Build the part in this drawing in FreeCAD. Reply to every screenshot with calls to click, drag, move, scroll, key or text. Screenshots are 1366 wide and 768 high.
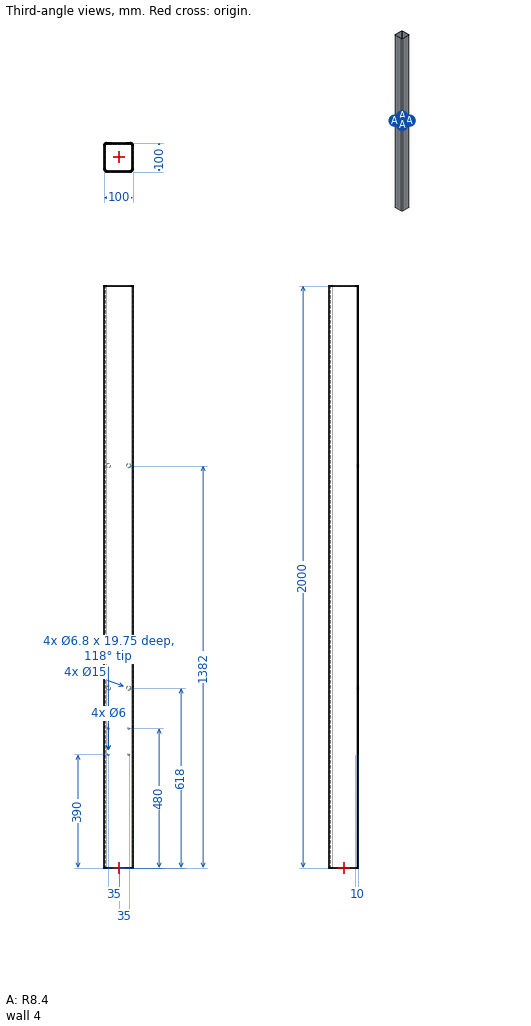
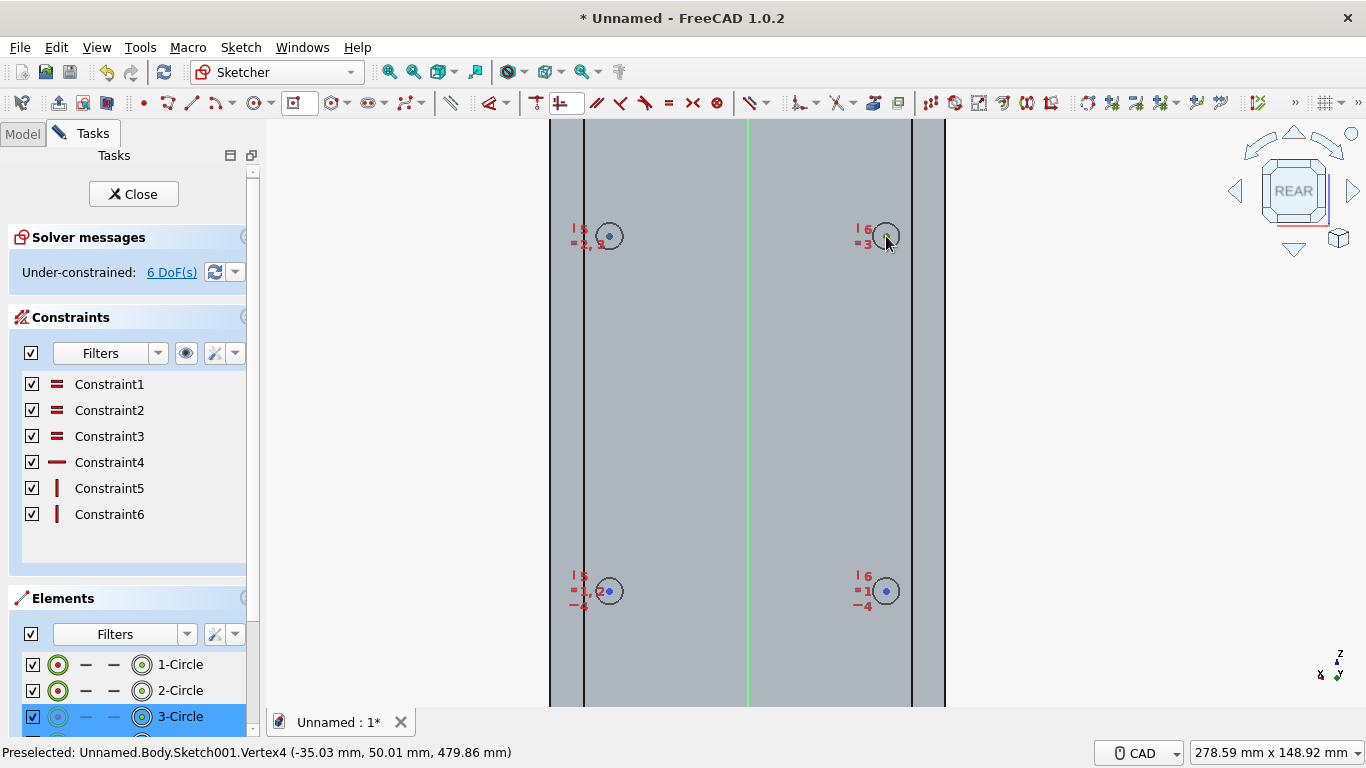
click(578, 104)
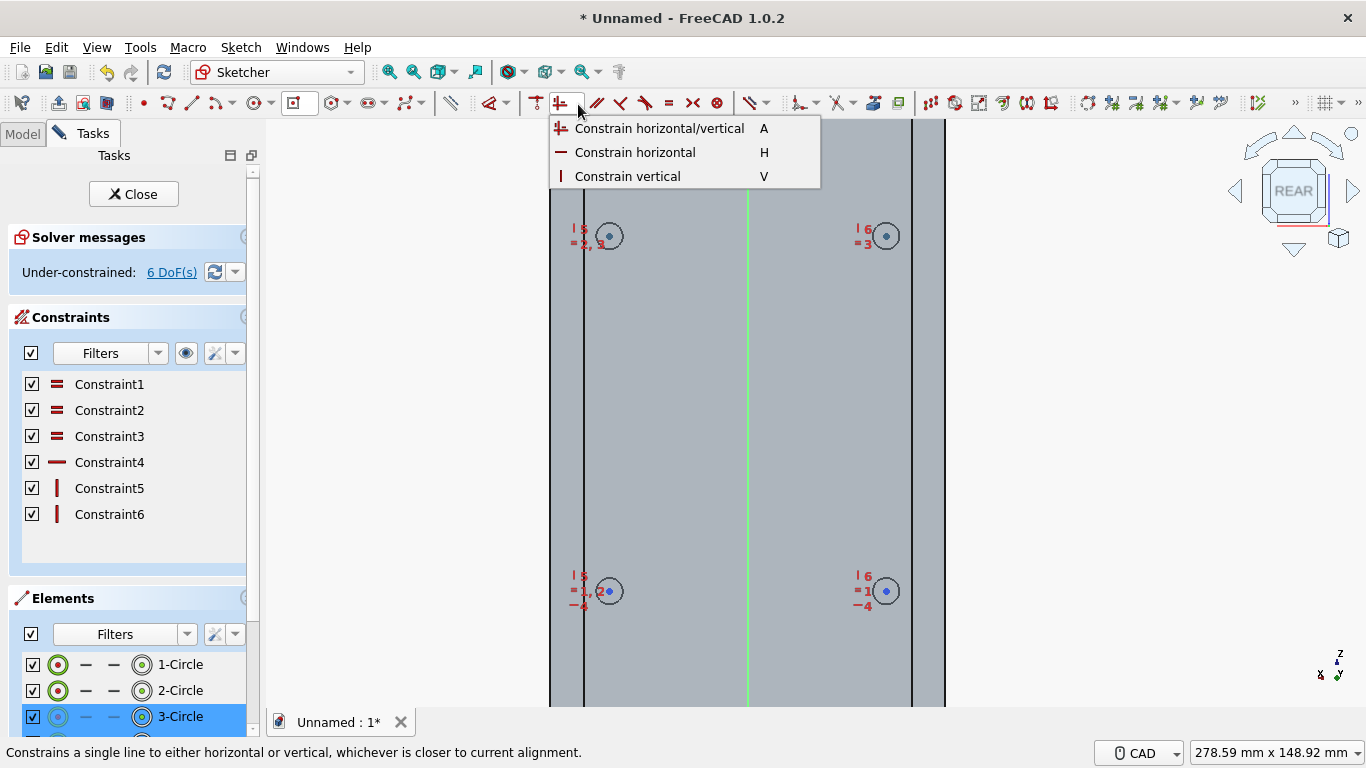
click(685, 152)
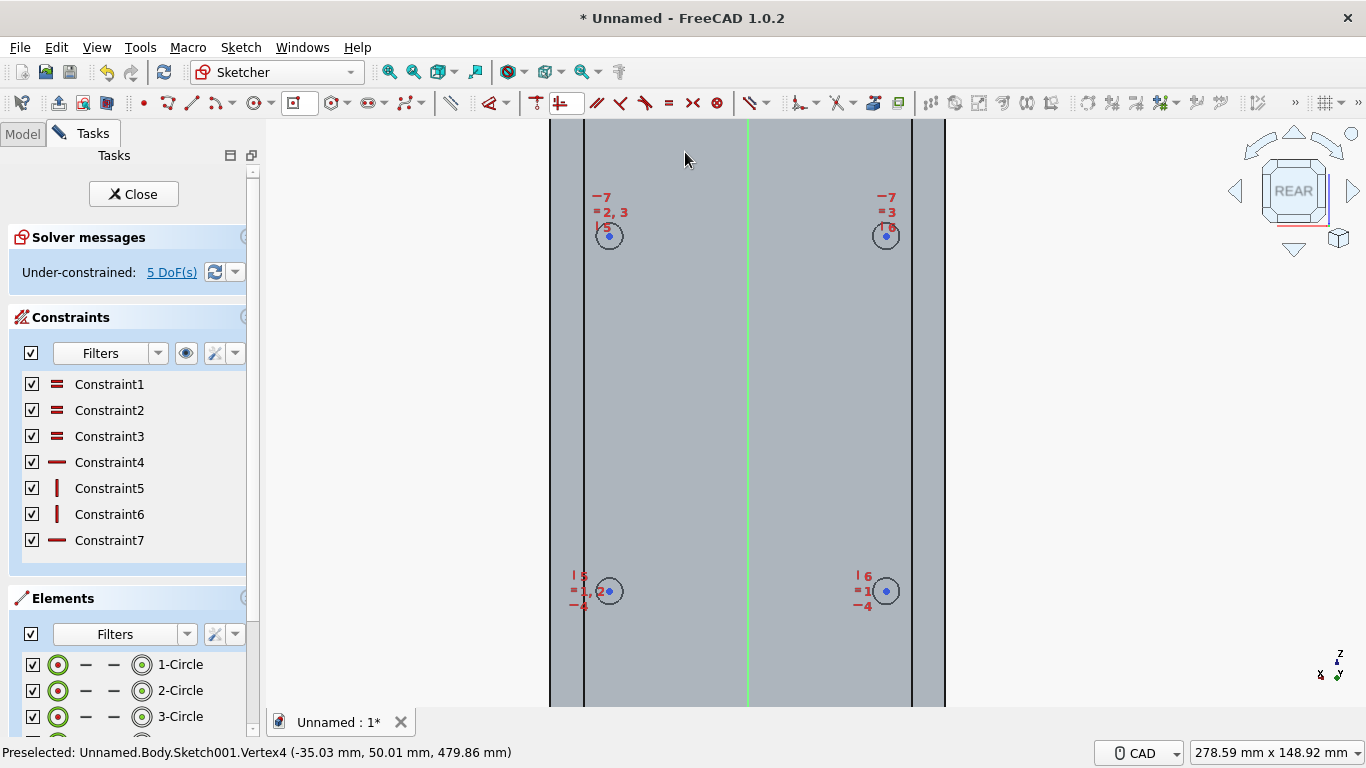
click(490, 104)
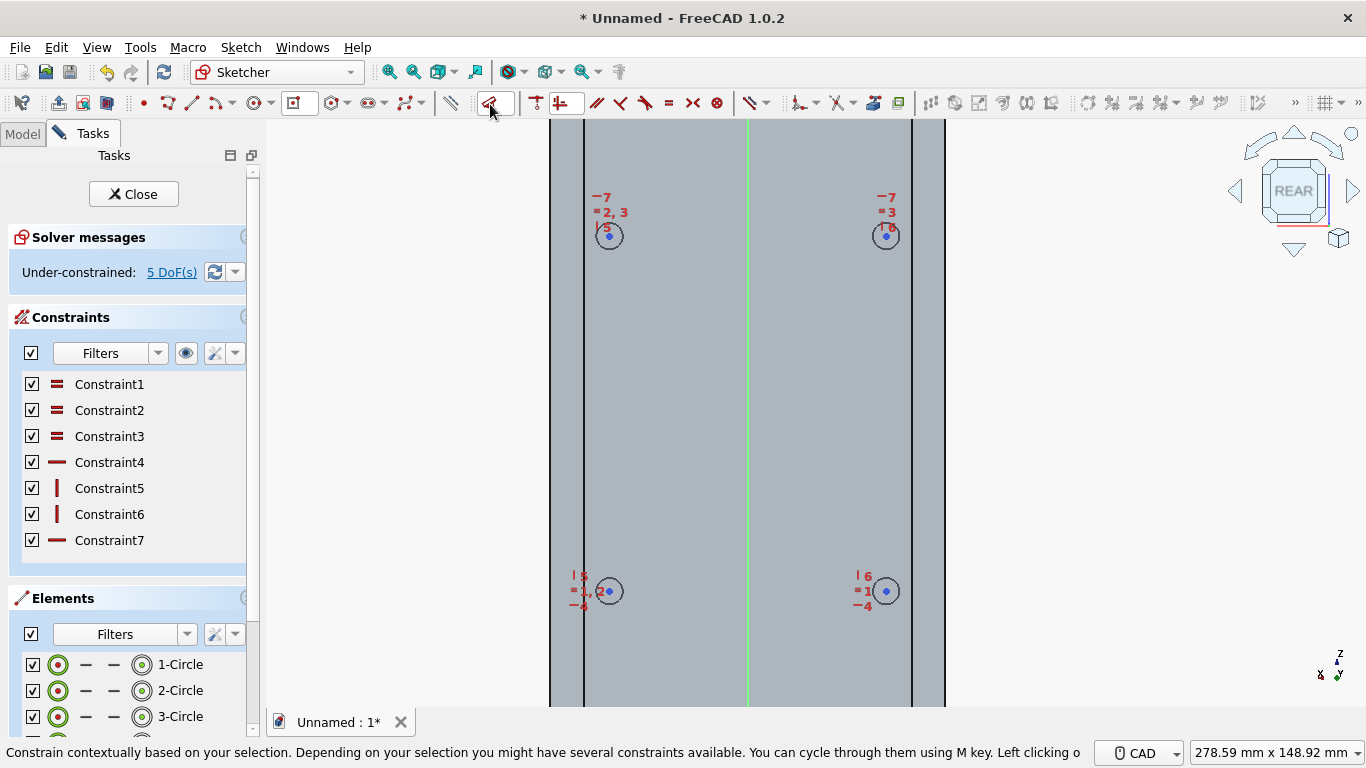
scroll(895, 582, up, 2)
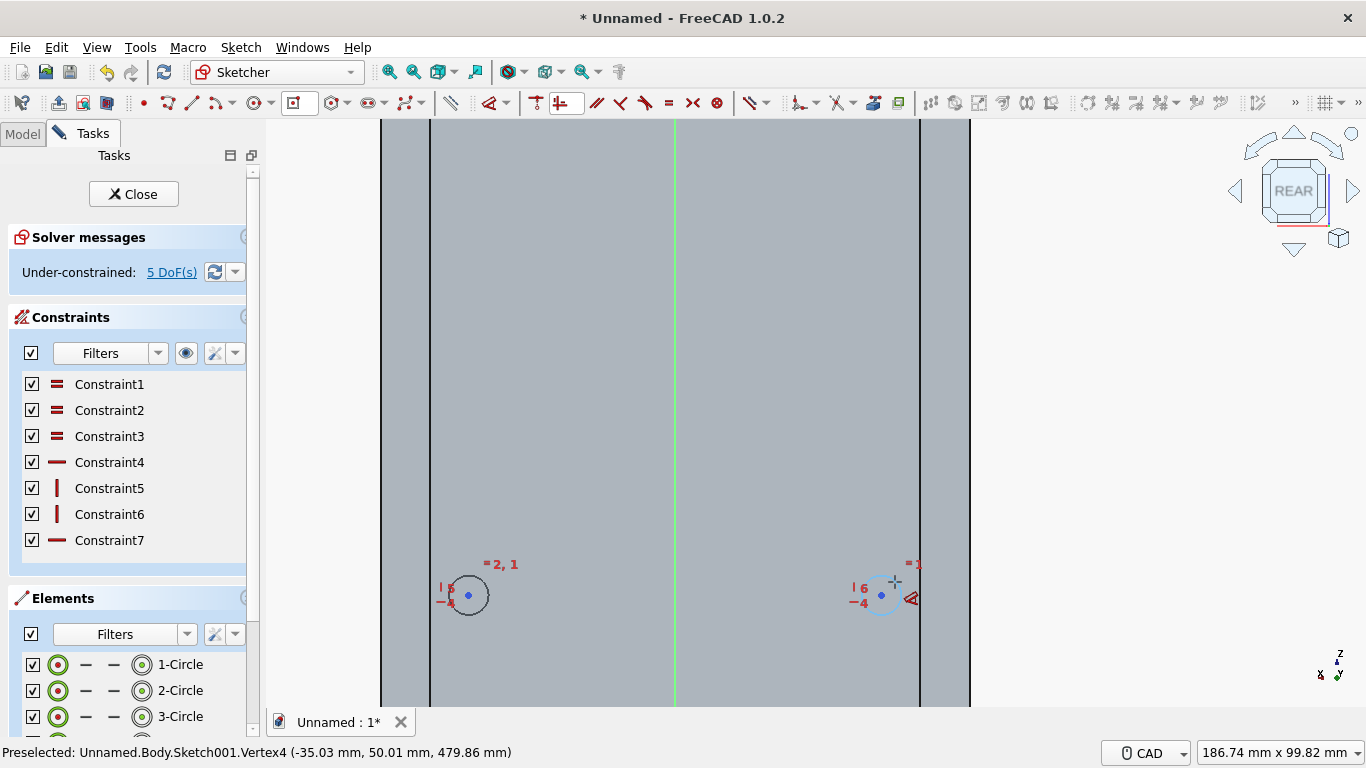
click(895, 581)
click(917, 558)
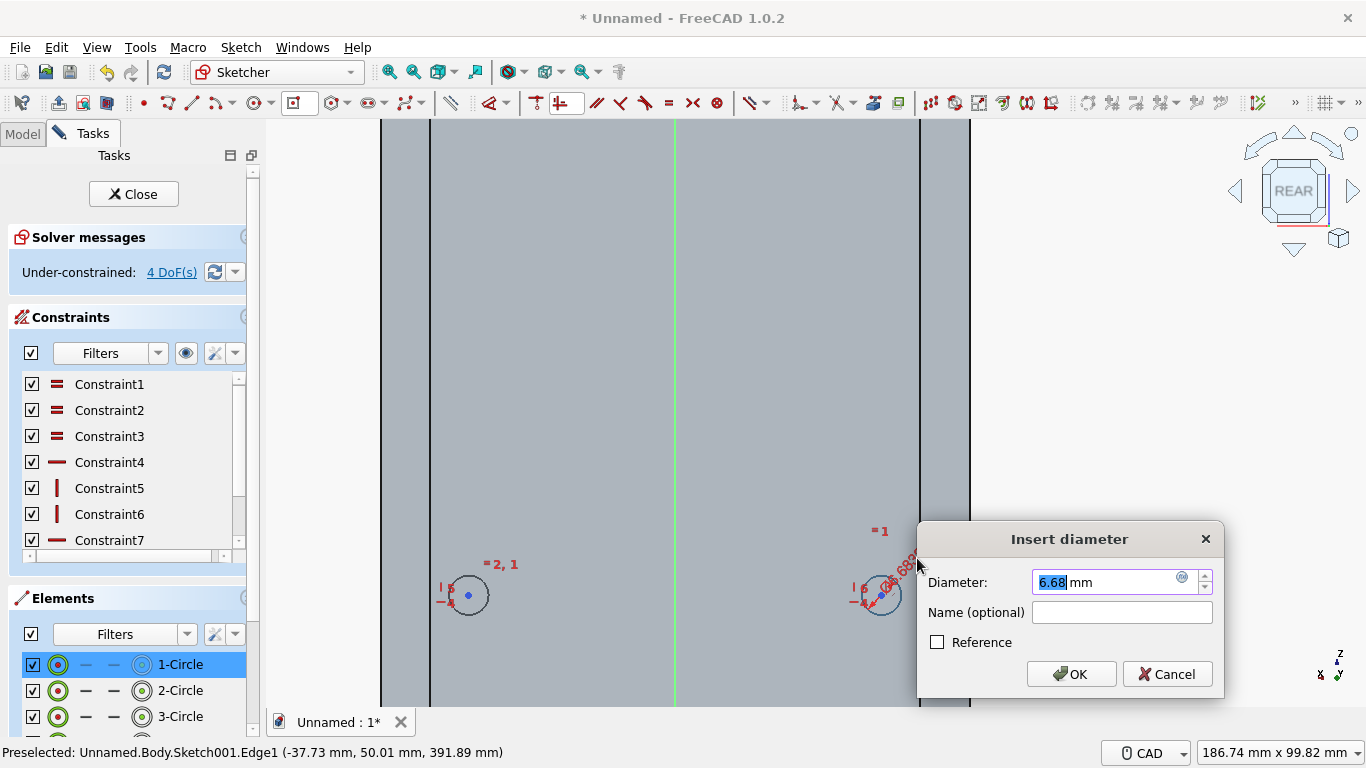
text(6.8)
key(Return)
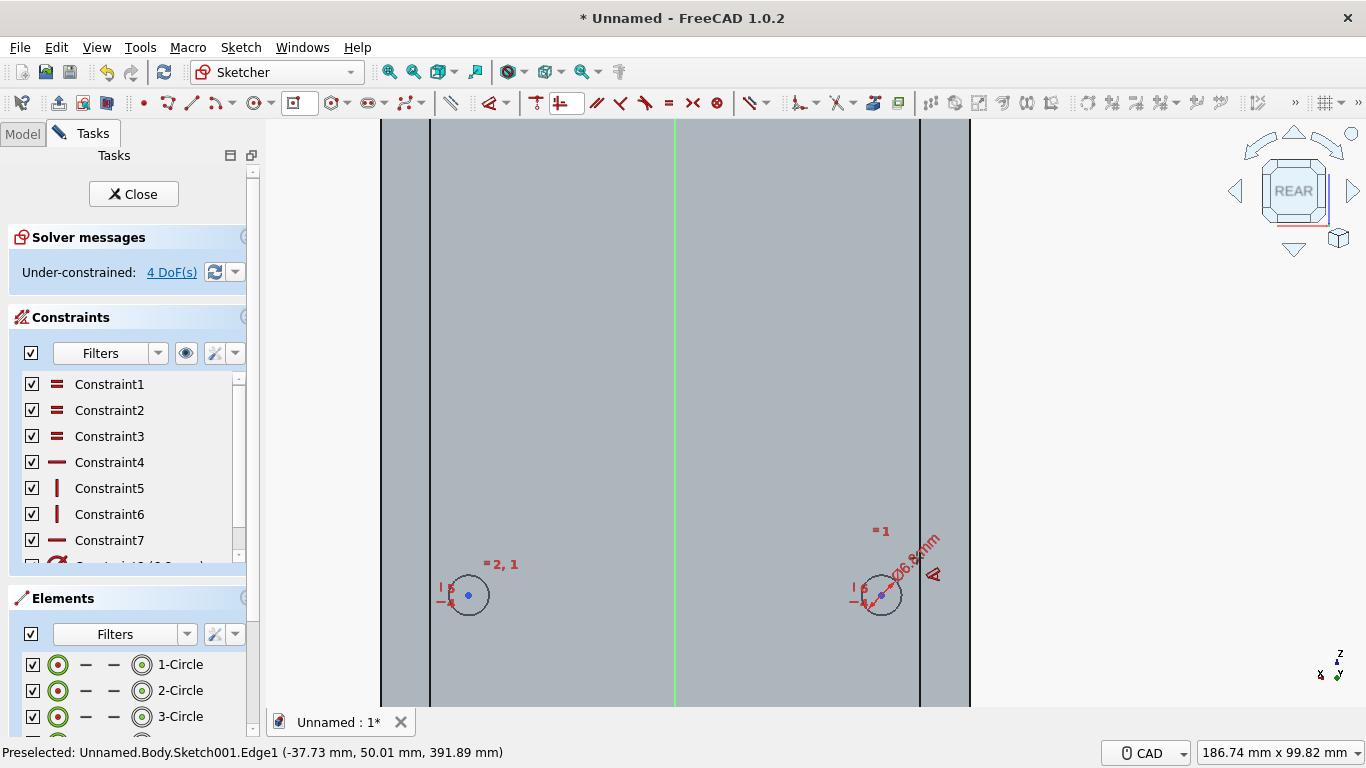
click(882, 595)
click(778, 561)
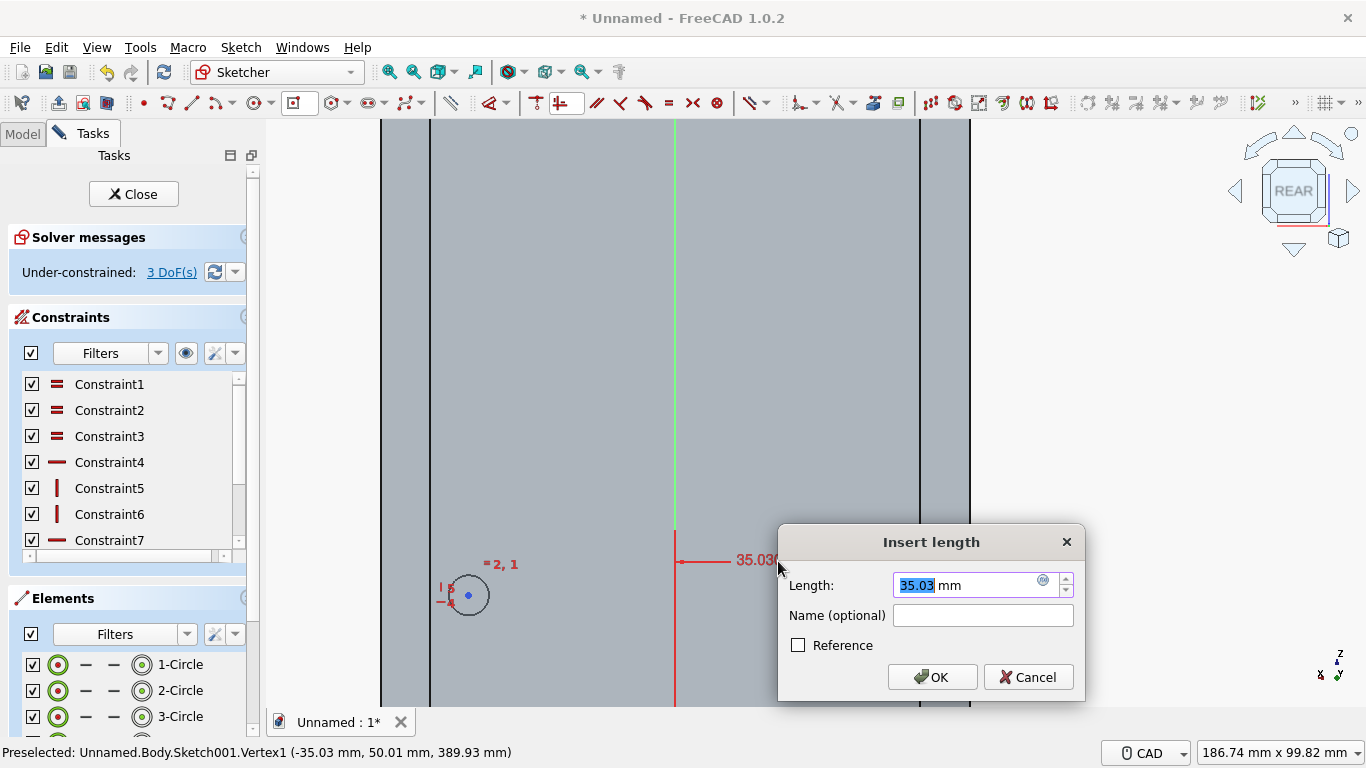
text(35)
key(Return)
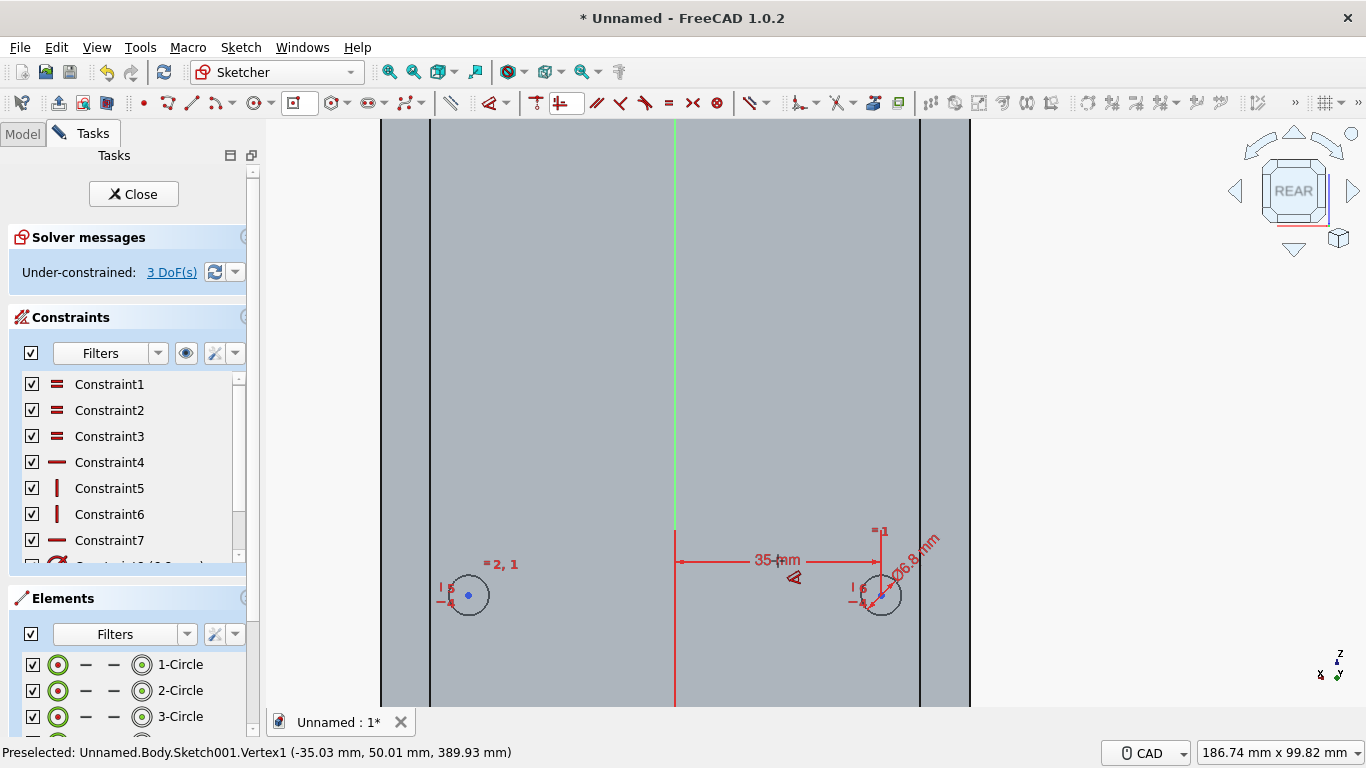
click(469, 595)
click(572, 561)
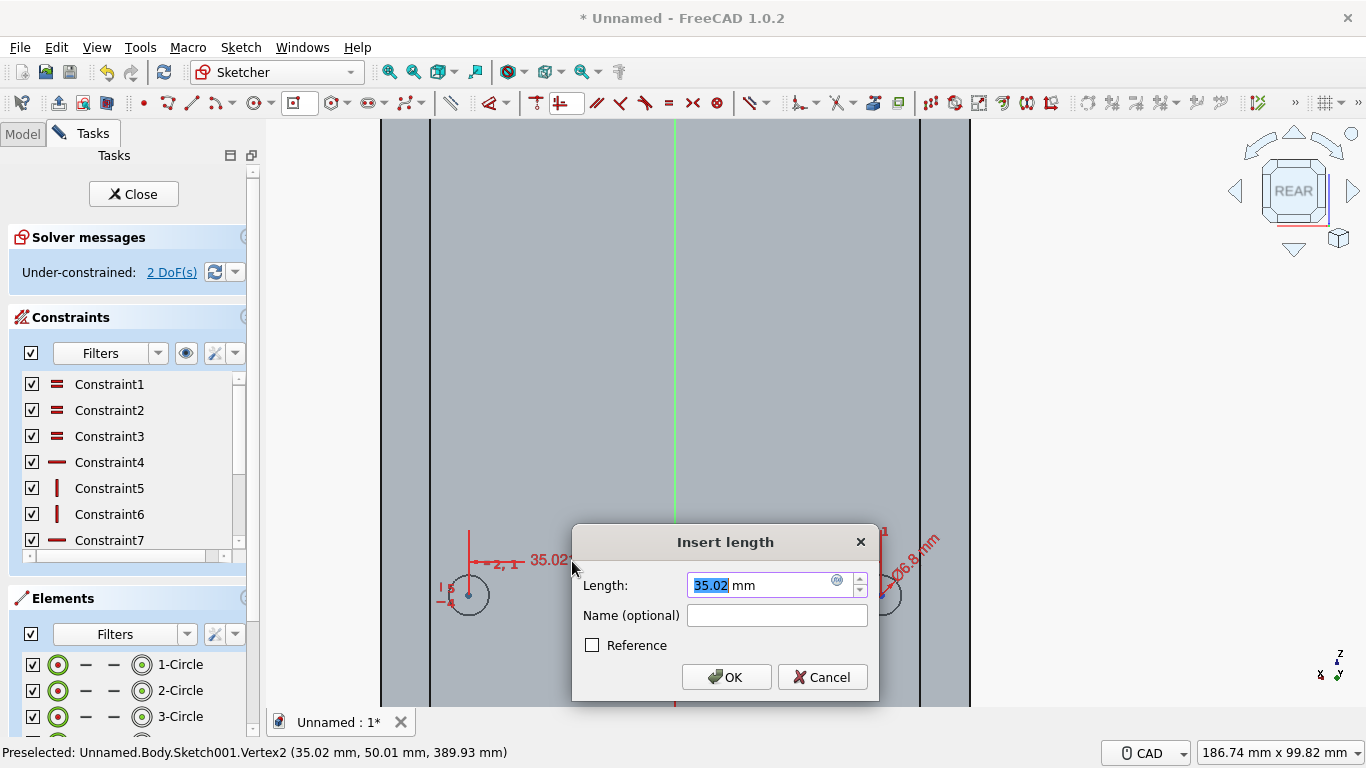
text(35)
key(Return)